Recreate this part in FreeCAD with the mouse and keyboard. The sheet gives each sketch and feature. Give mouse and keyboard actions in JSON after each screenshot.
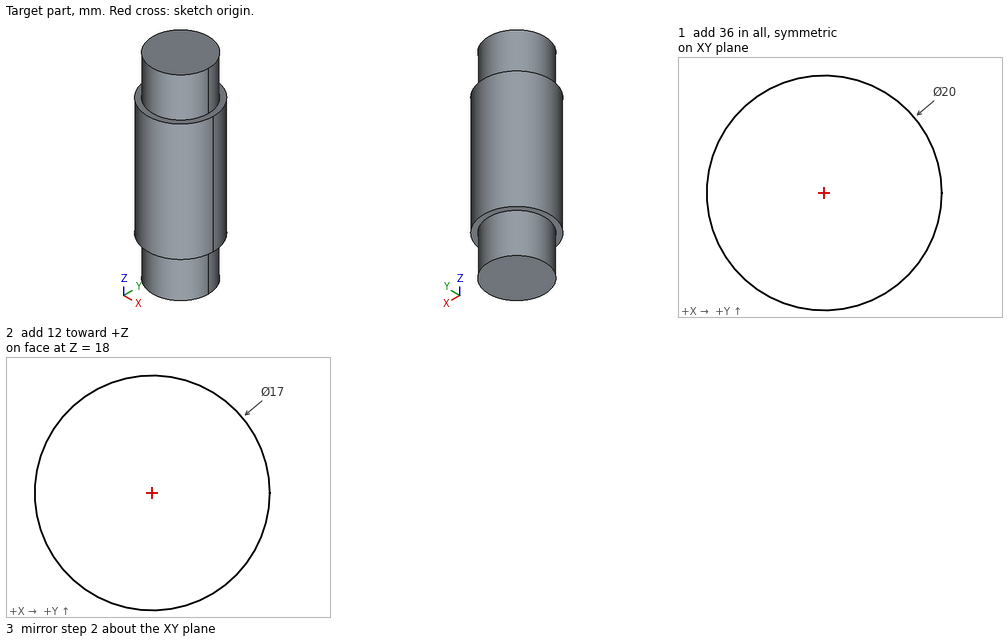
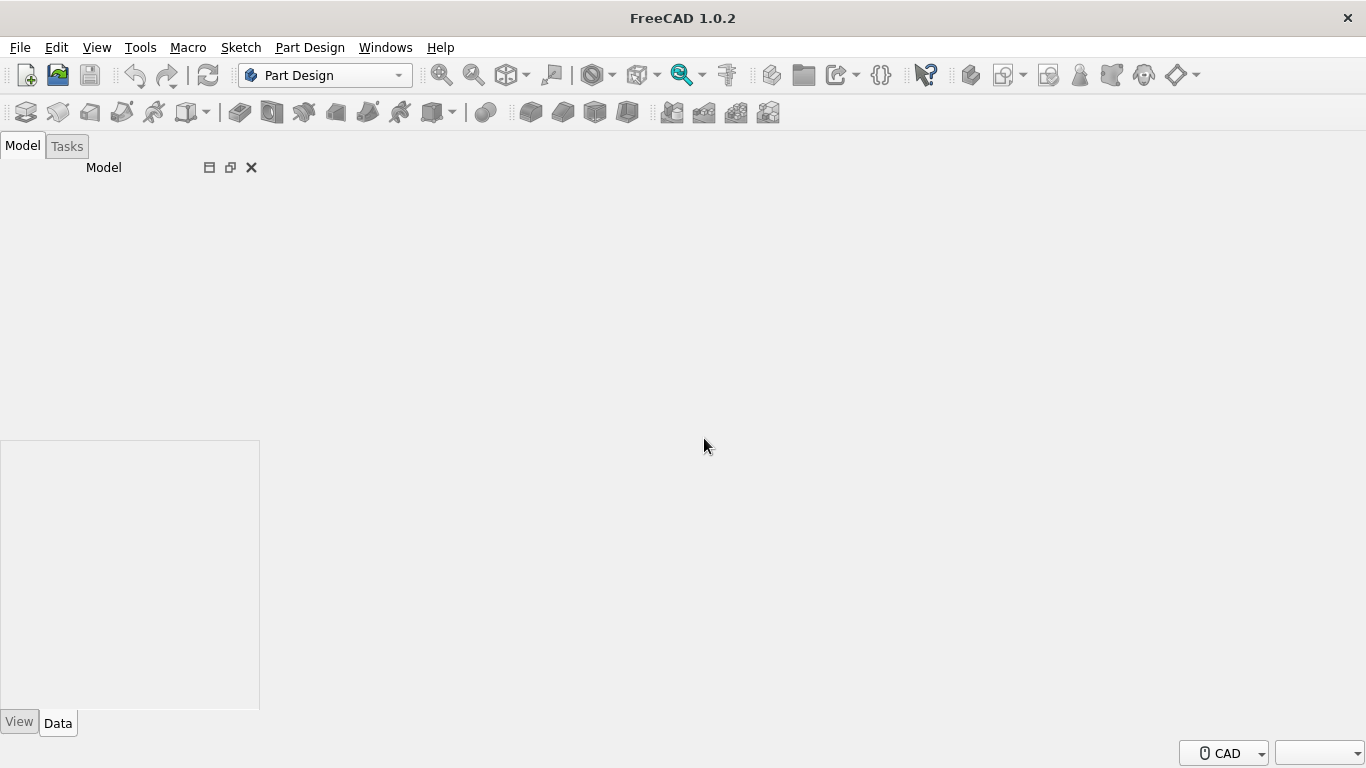
{"action": "left_click", "coordinate": [26, 76]}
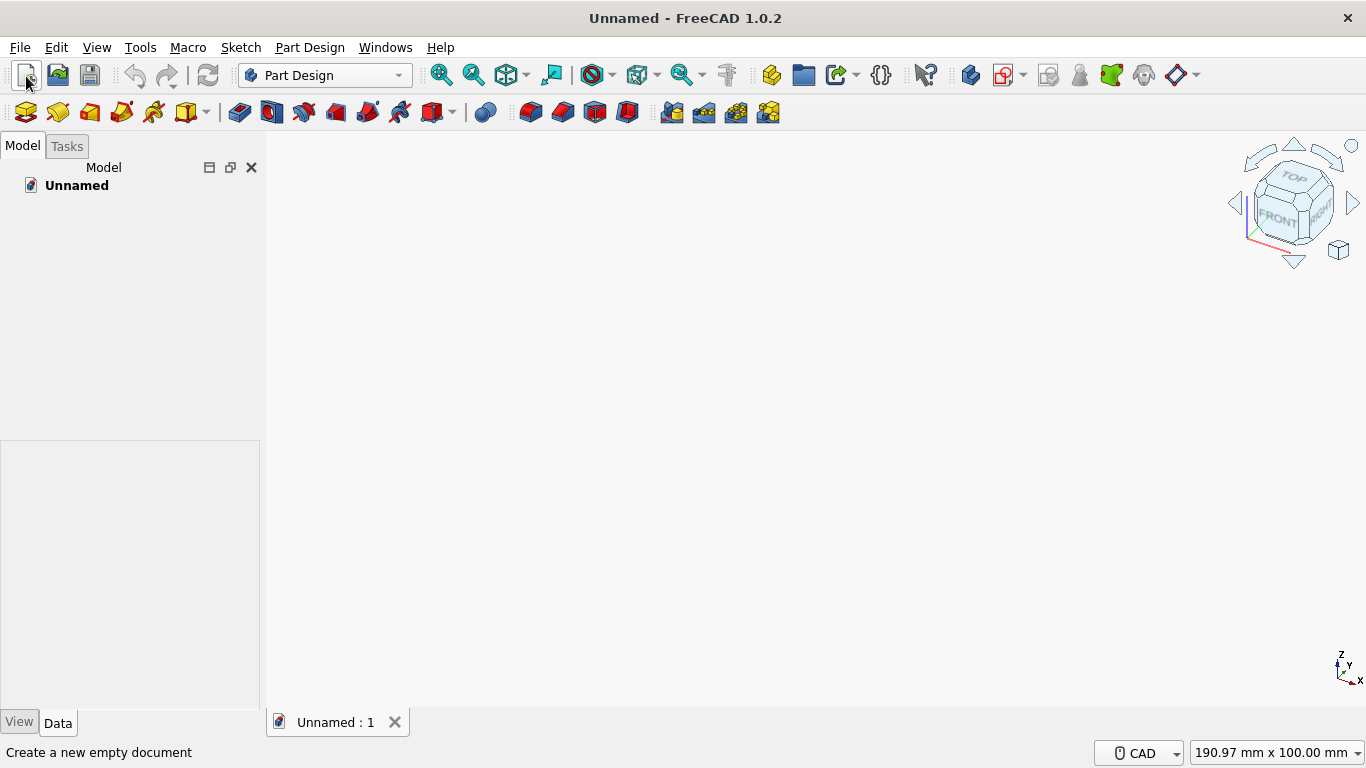
{"action": "left_click", "coordinate": [1004, 76]}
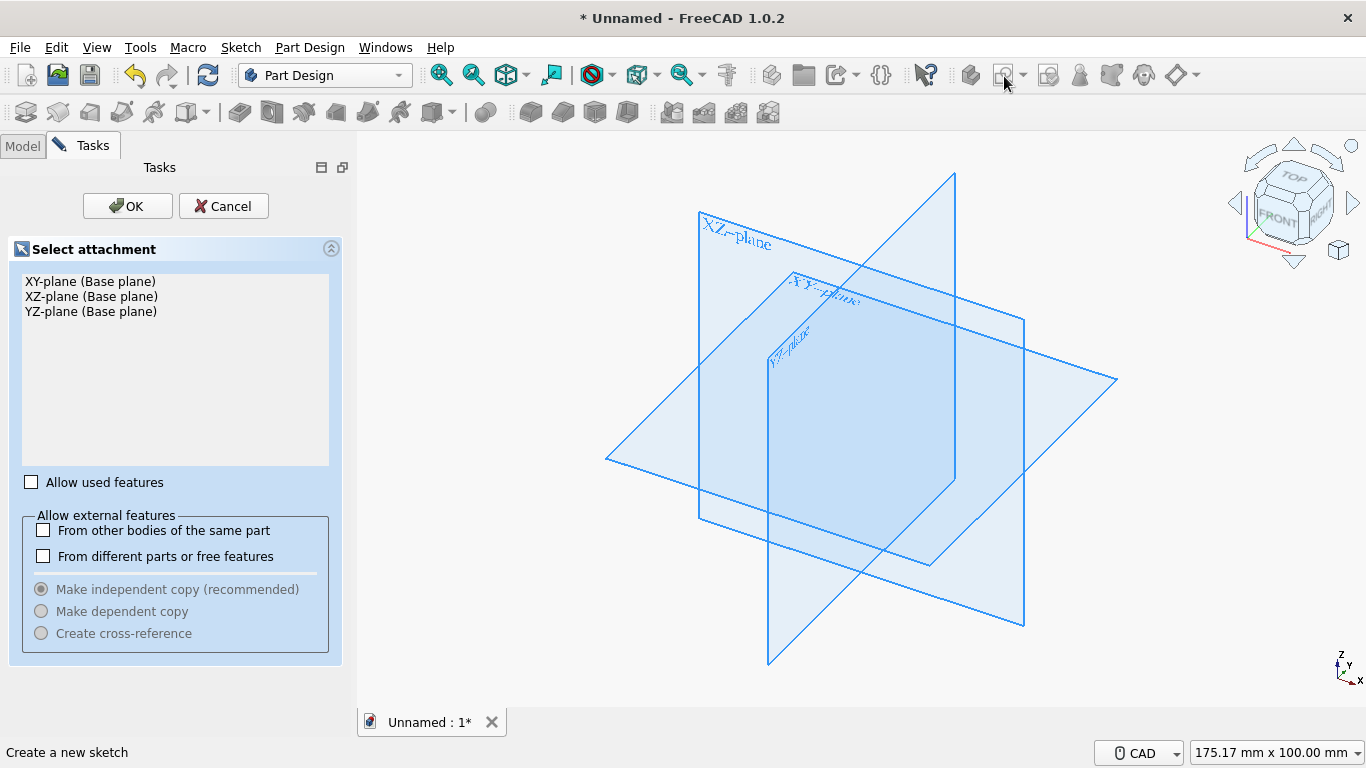
{"action": "left_click", "coordinate": [82, 282]}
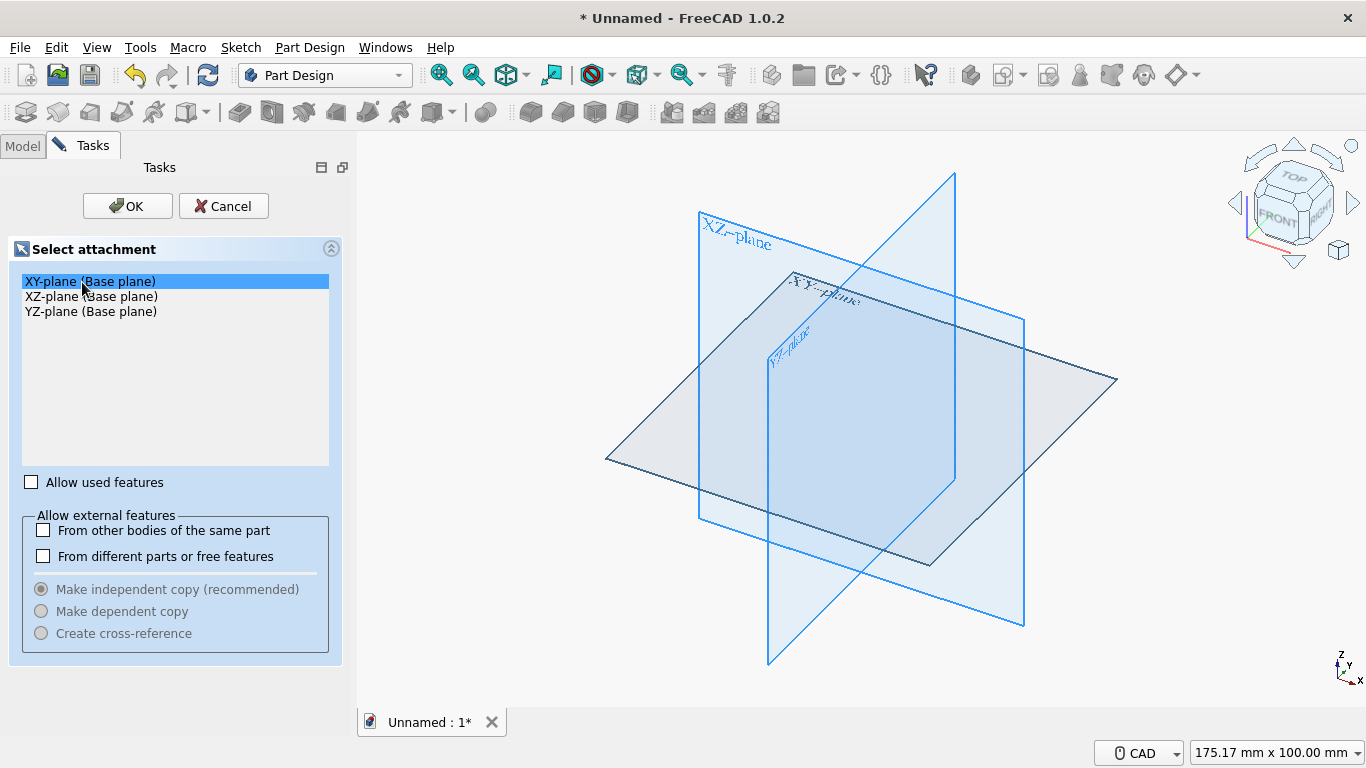
{"action": "left_click", "coordinate": [128, 206]}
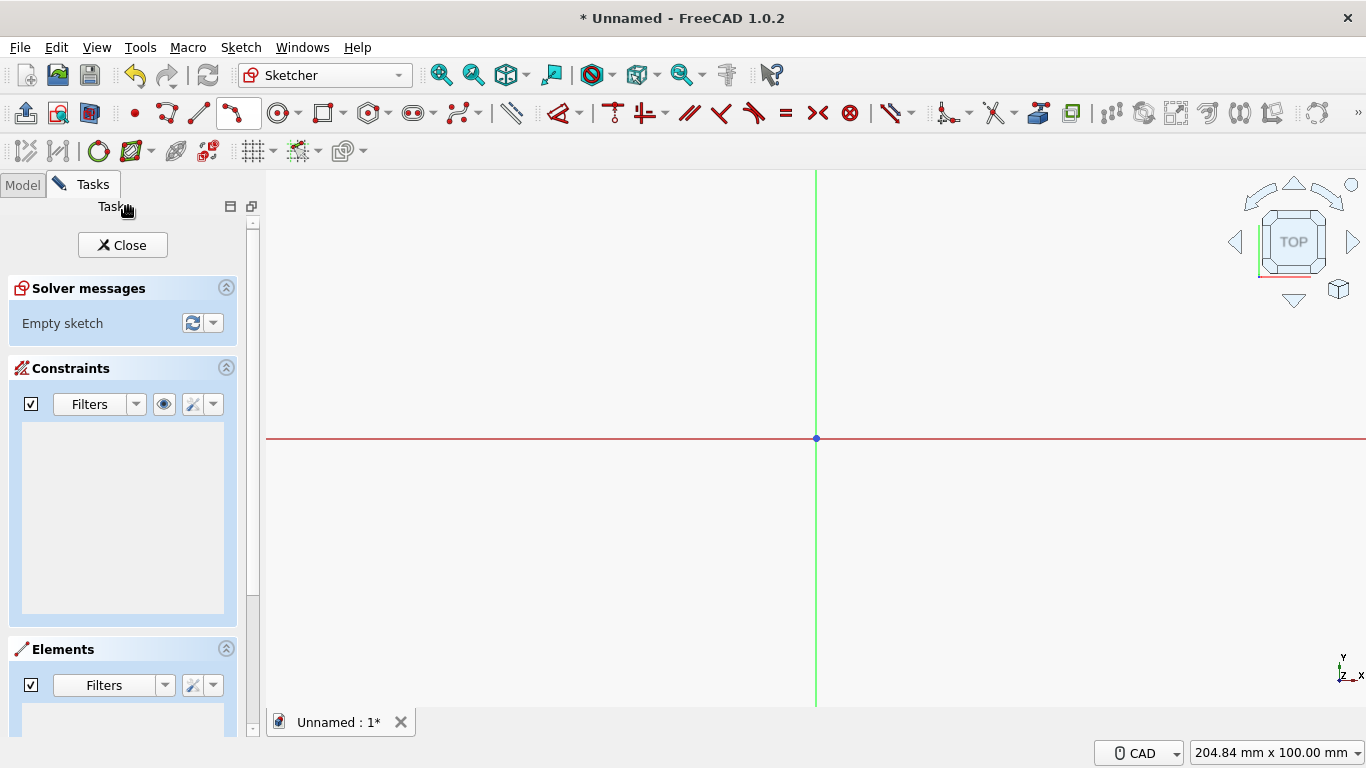
{"action": "scroll", "coordinate": [846, 438], "scroll_direction": "up", "scroll_amount": 6}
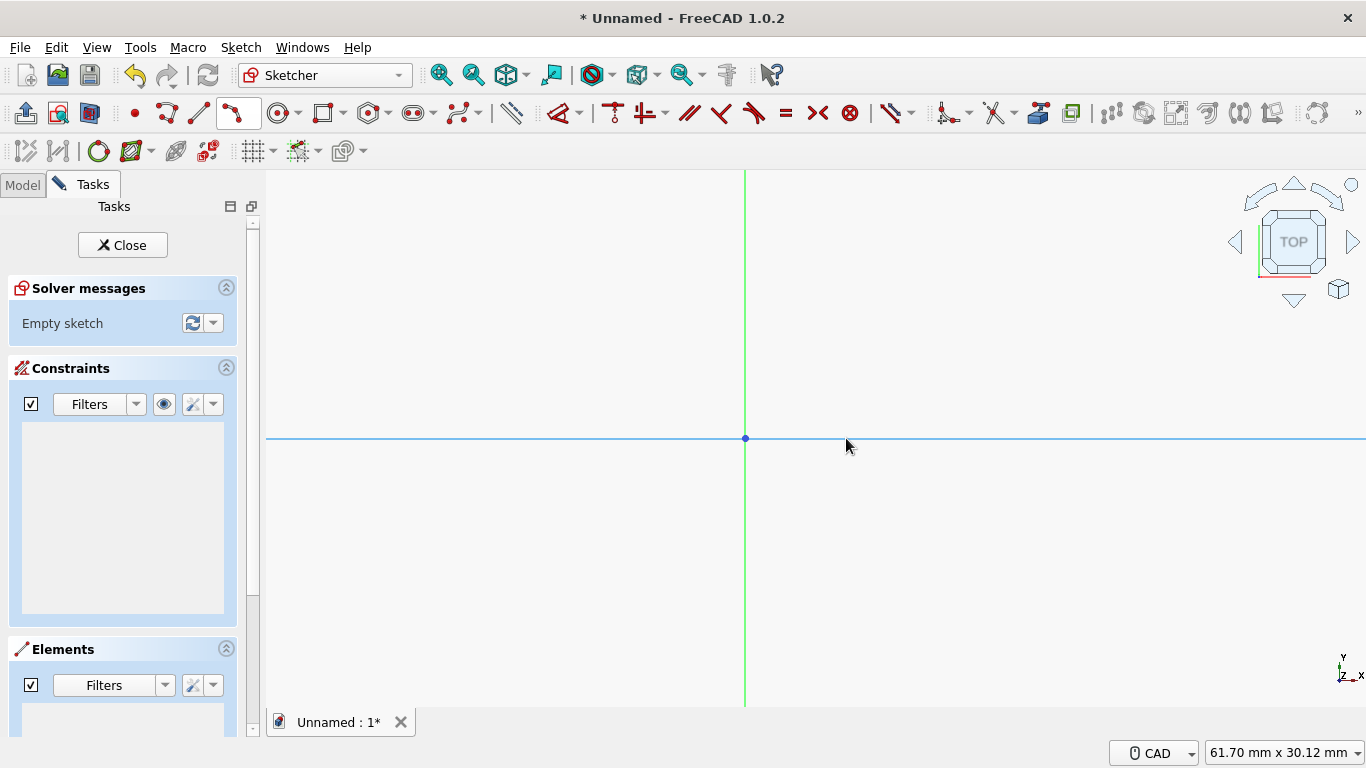
{"action": "left_click", "coordinate": [278, 114]}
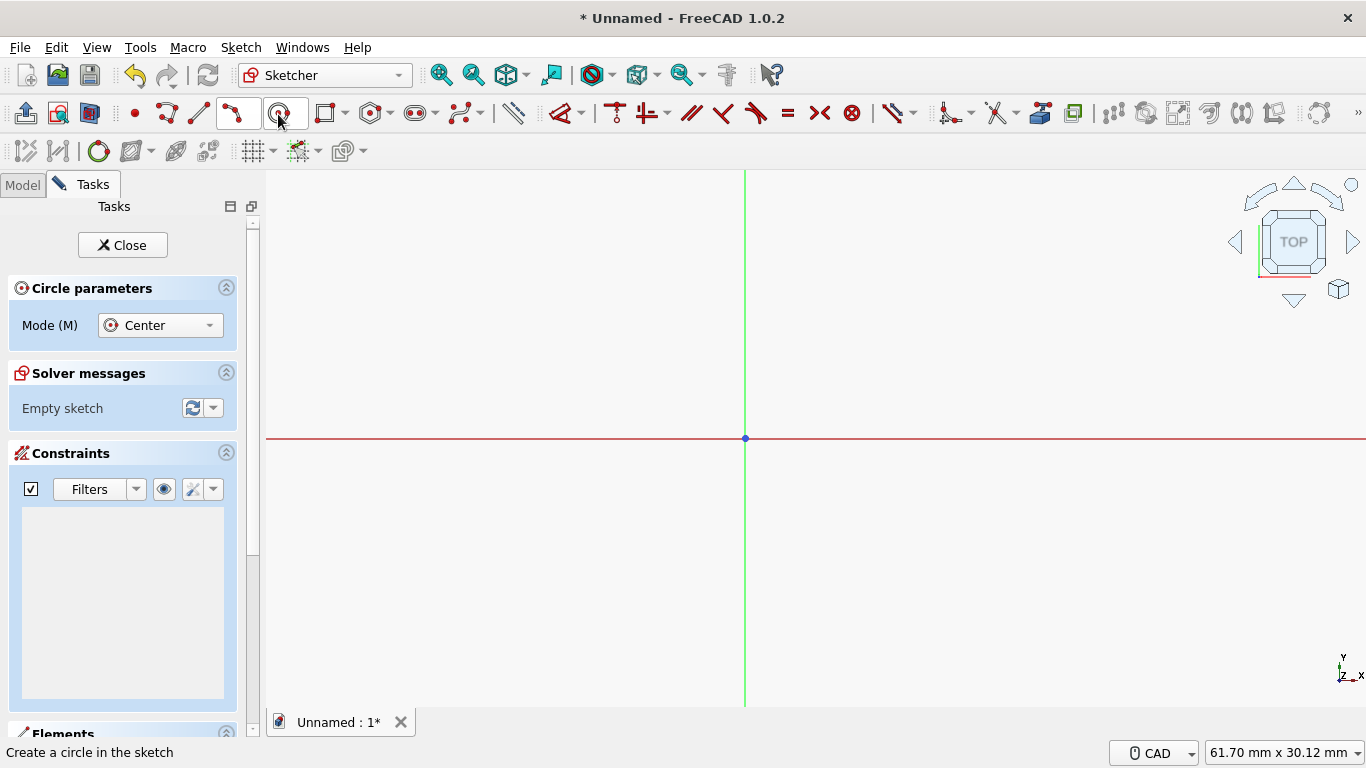
{"action": "left_click", "coordinate": [745, 438]}
{"action": "left_click", "coordinate": [871, 312]}
{"action": "key", "text": "Escape"}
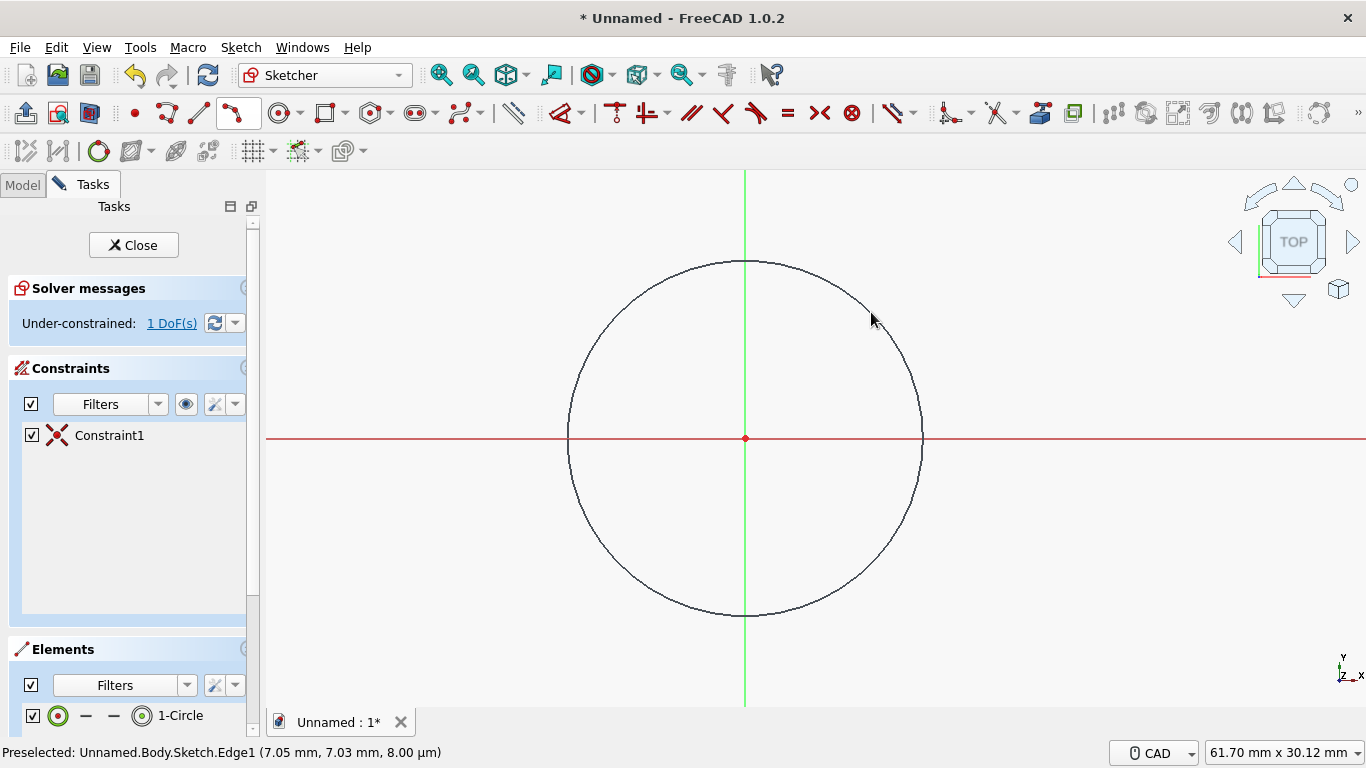
{"action": "left_click", "coordinate": [560, 114]}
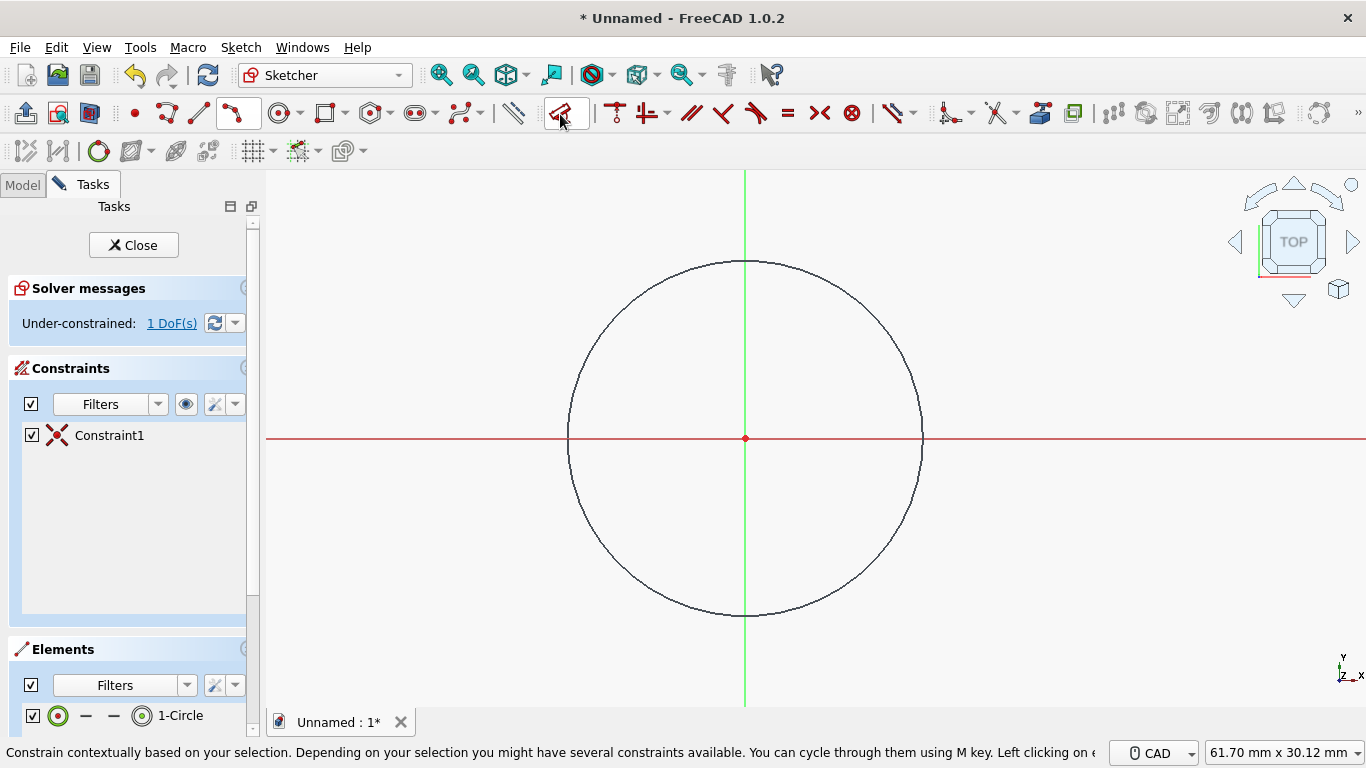
{"action": "left_click", "coordinate": [870, 312]}
{"action": "left_click", "coordinate": [892, 289]}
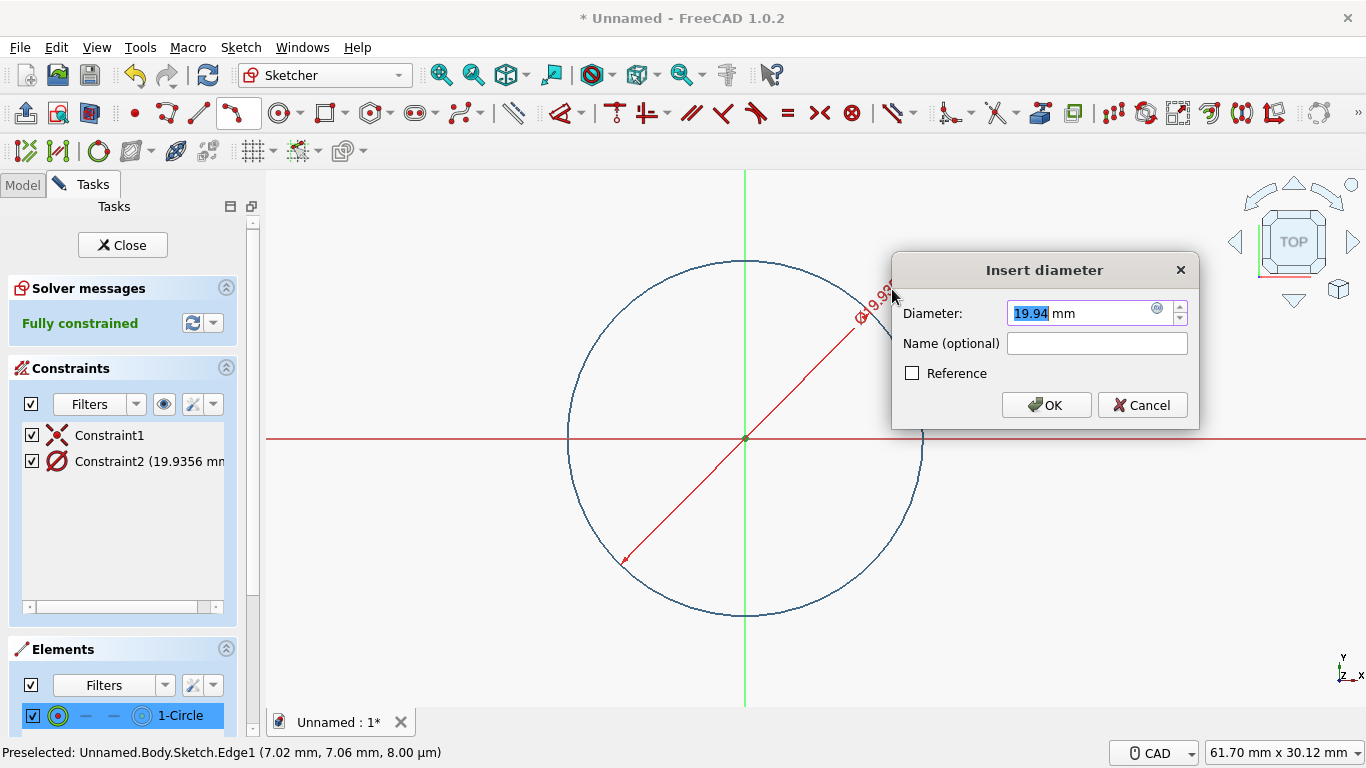
{"action": "type", "text": "20"}
{"action": "key", "text": "Return"}
{"action": "key", "text": "Escape"}